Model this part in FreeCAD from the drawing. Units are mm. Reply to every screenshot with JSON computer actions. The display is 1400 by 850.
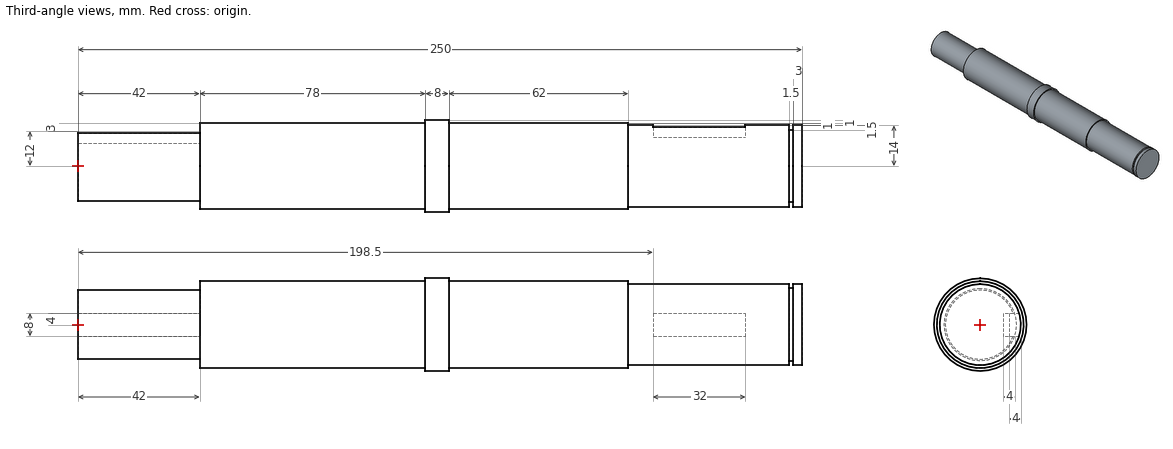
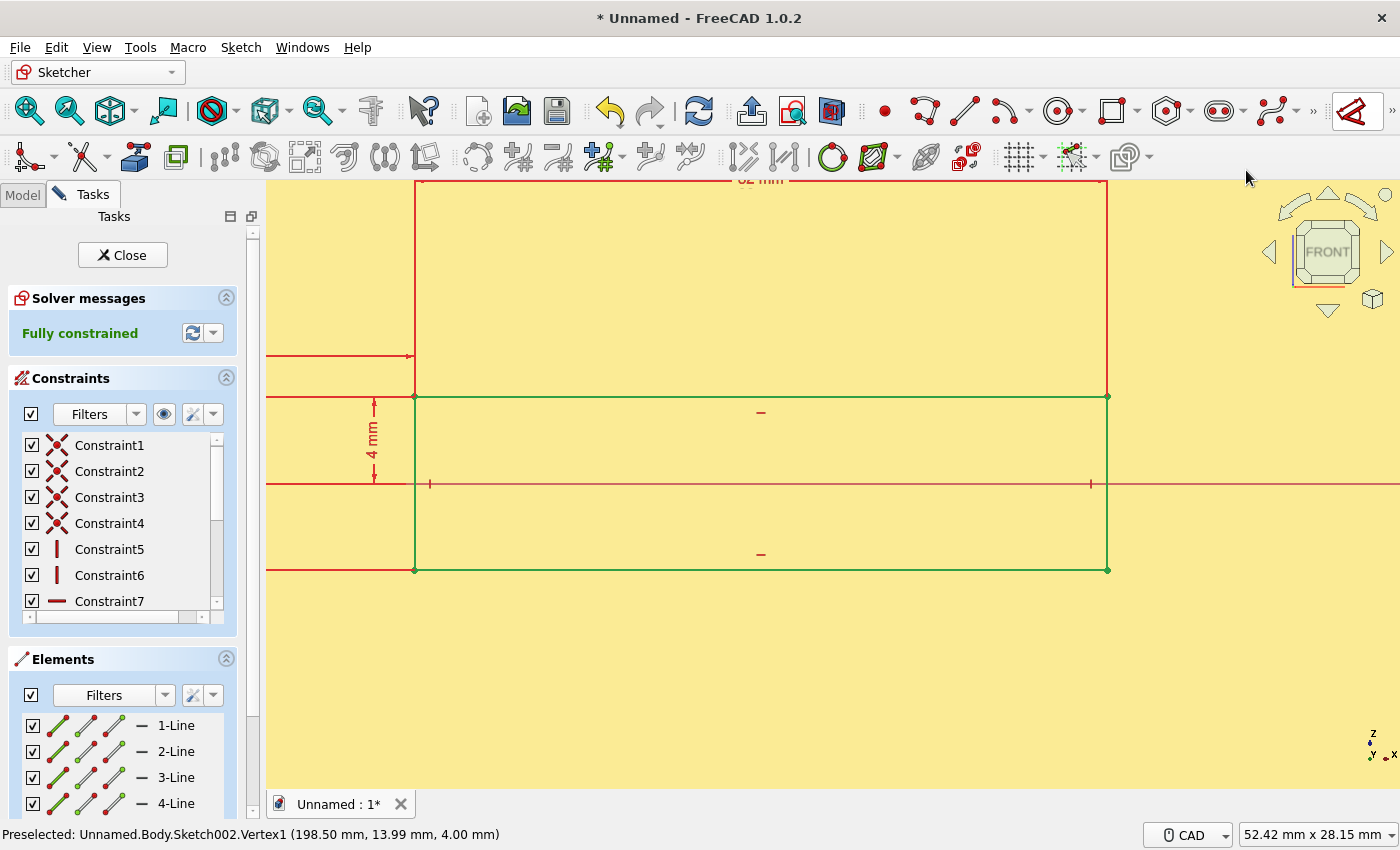
{"action": "left_click", "coordinate": [123, 255]}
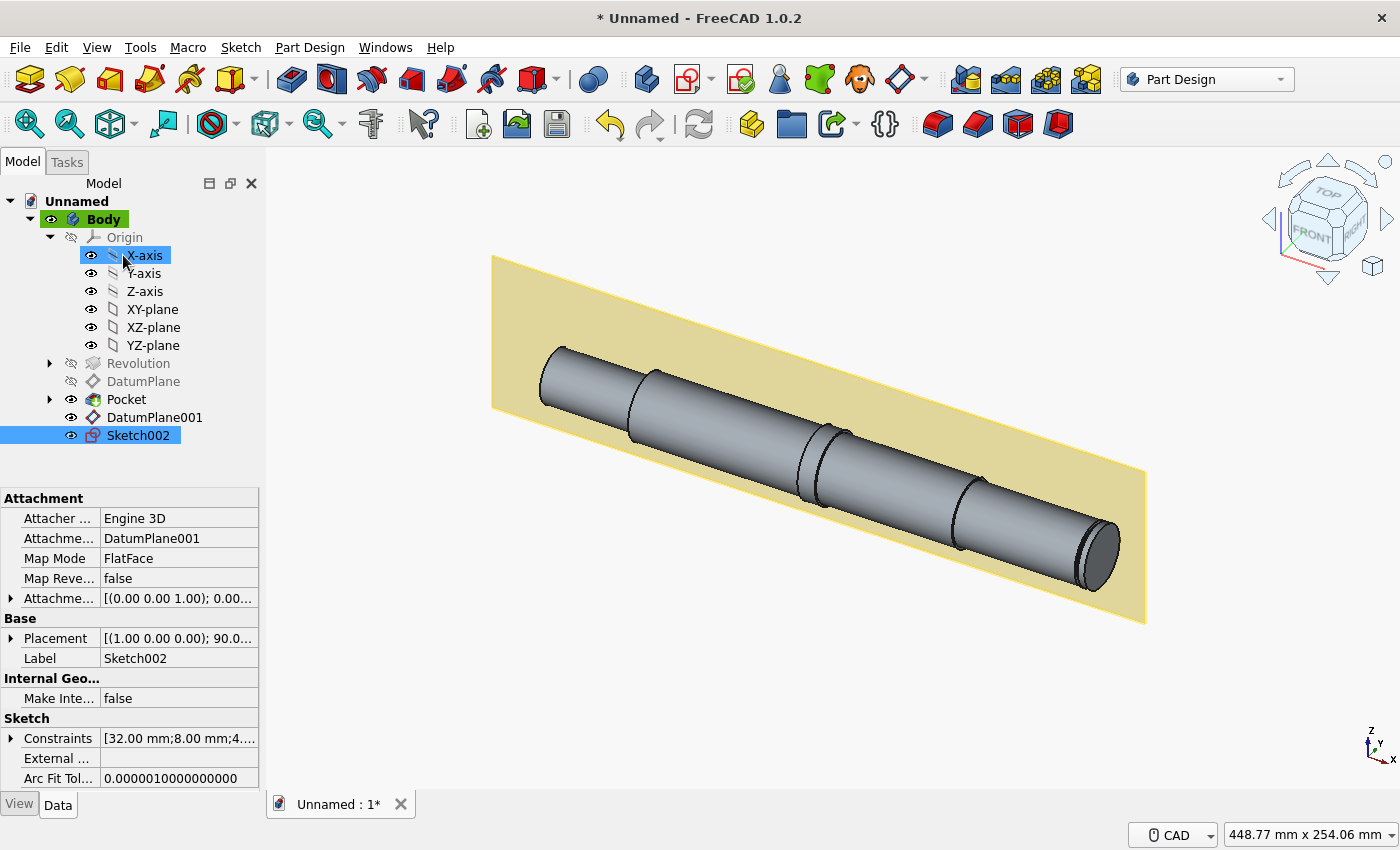
{"action": "left_click", "coordinate": [292, 80]}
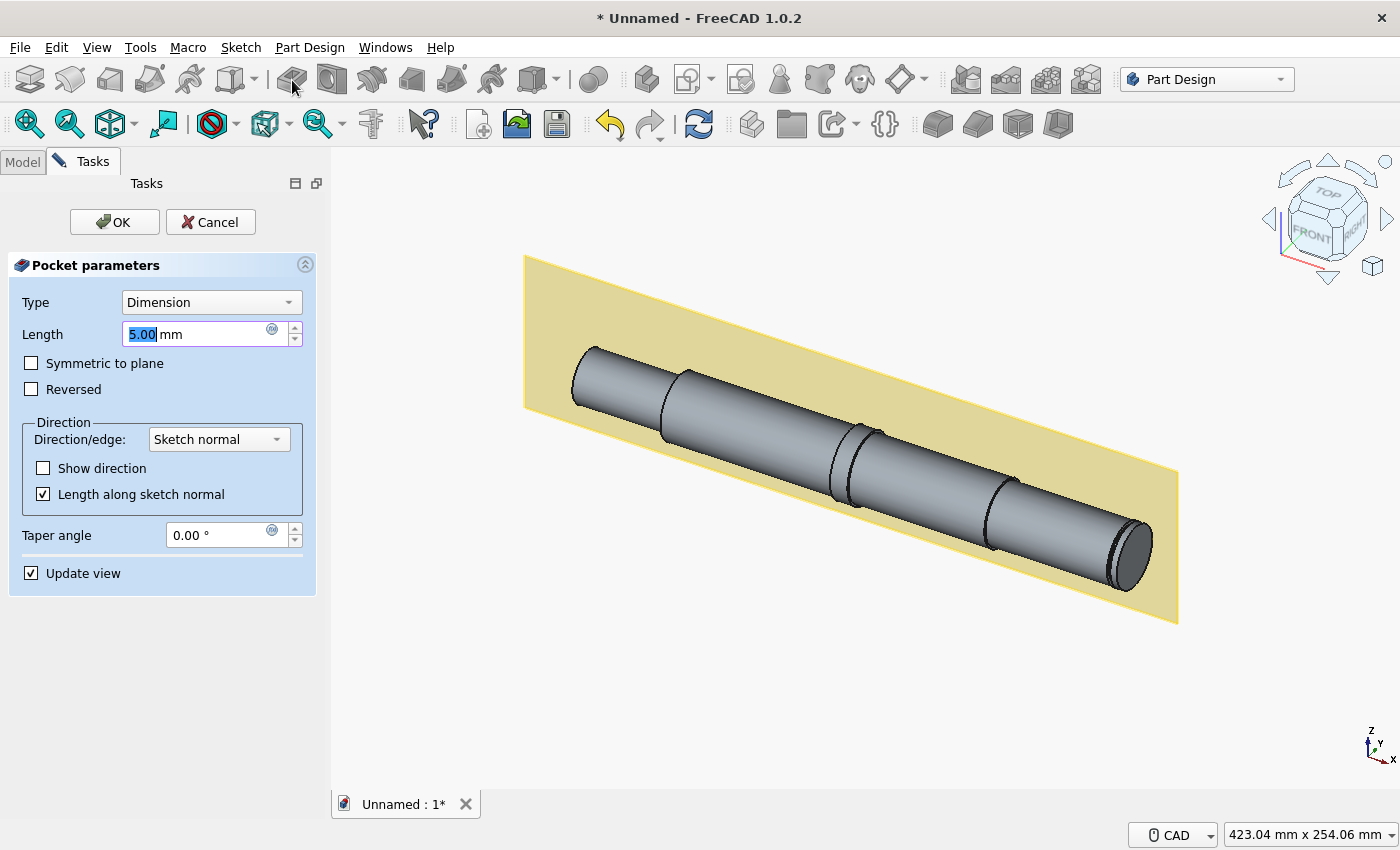
{"action": "type", "text": "4"}
{"action": "key", "text": "Tab"}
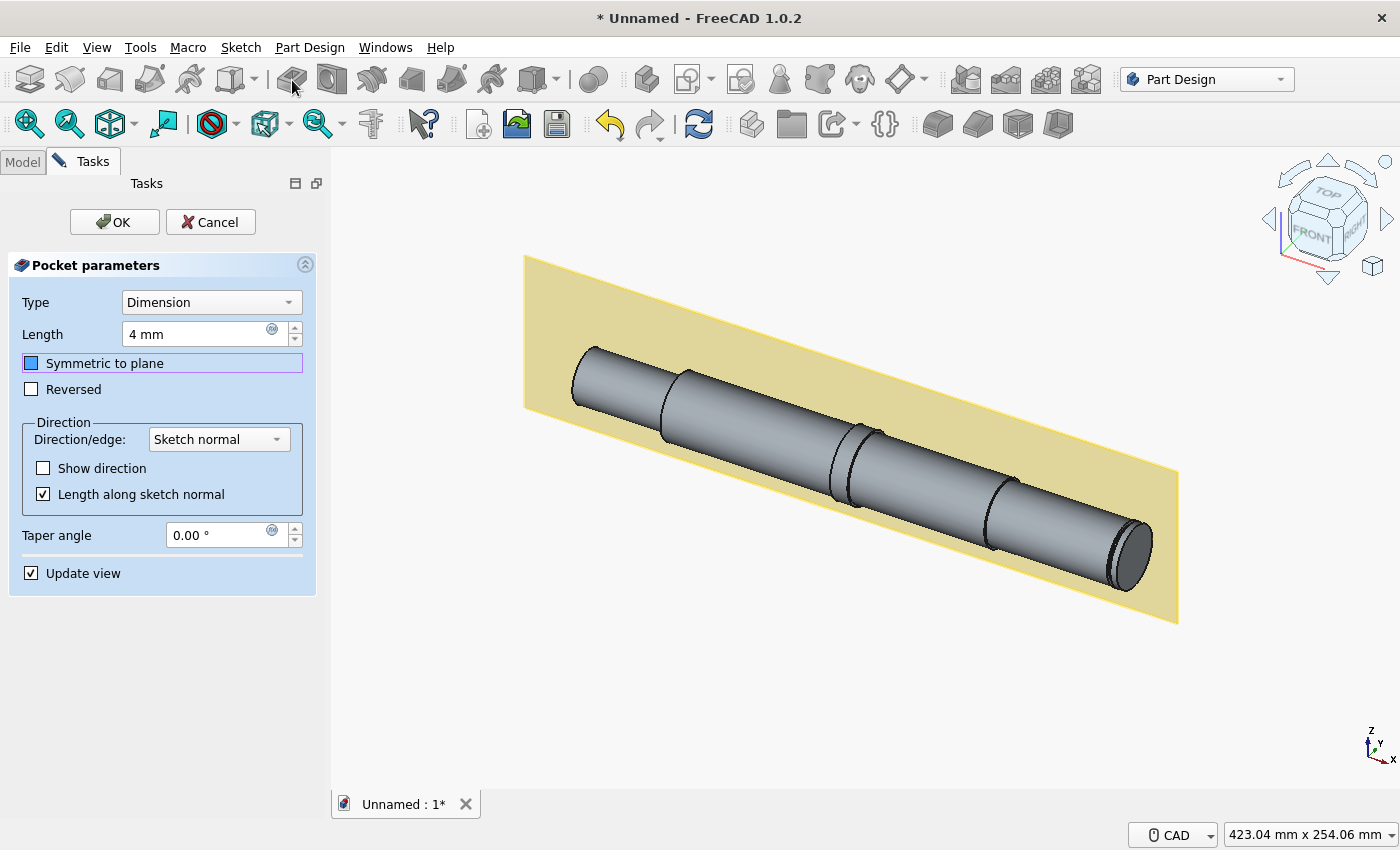
{"action": "left_click", "coordinate": [30, 389]}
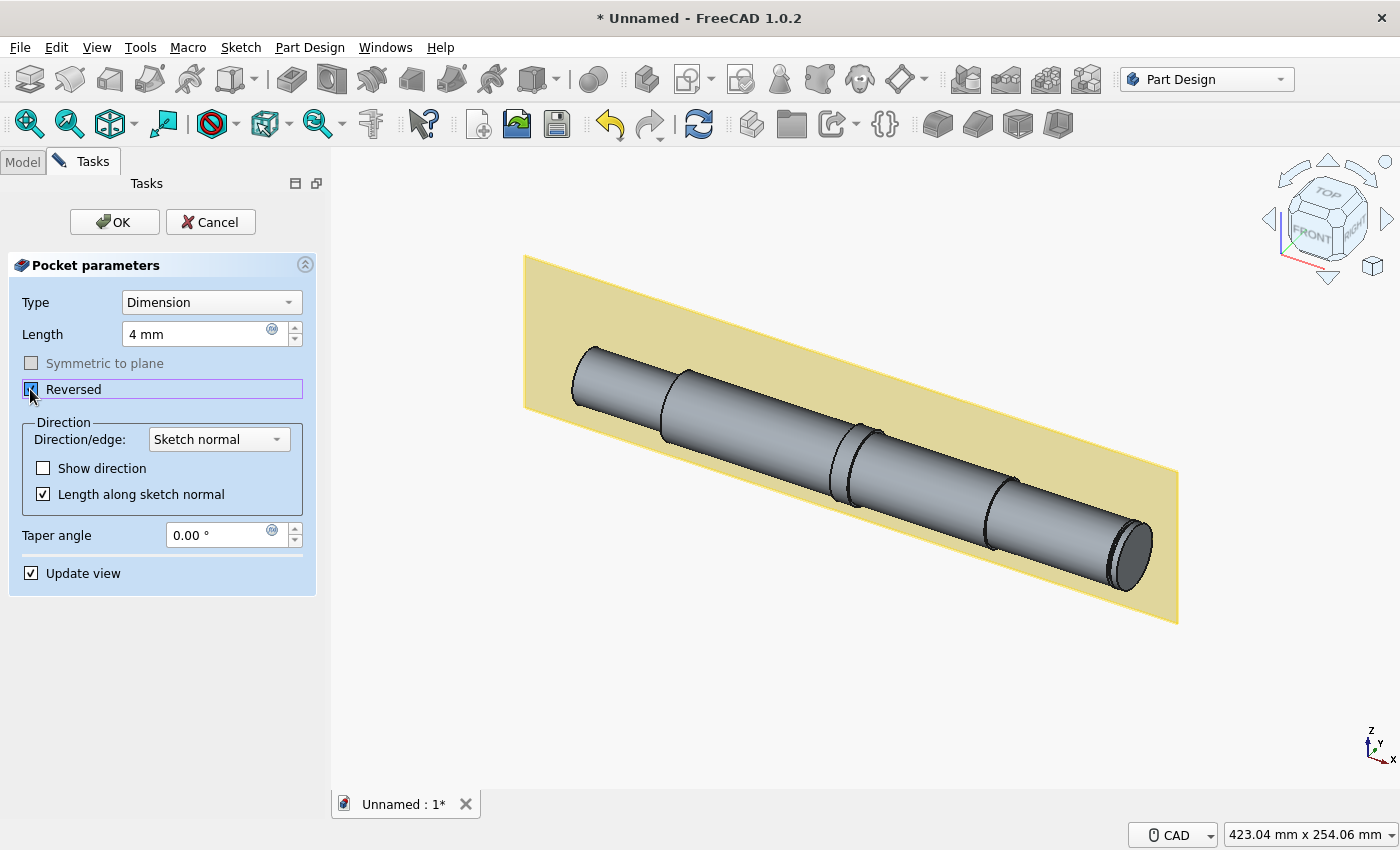
{"action": "left_click", "coordinate": [115, 222]}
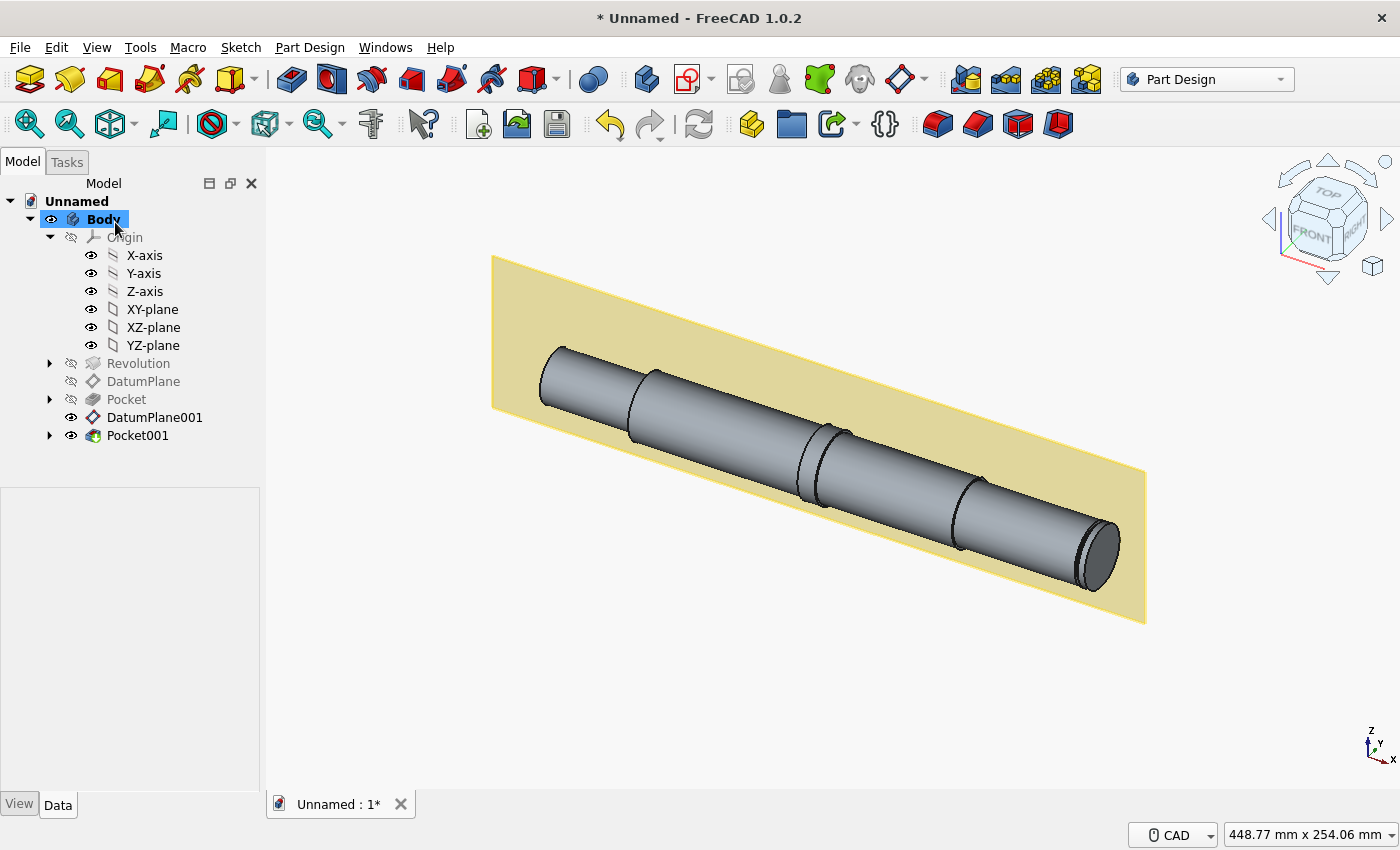
{"action": "left_click", "coordinate": [116, 417]}
{"action": "key", "text": "space"}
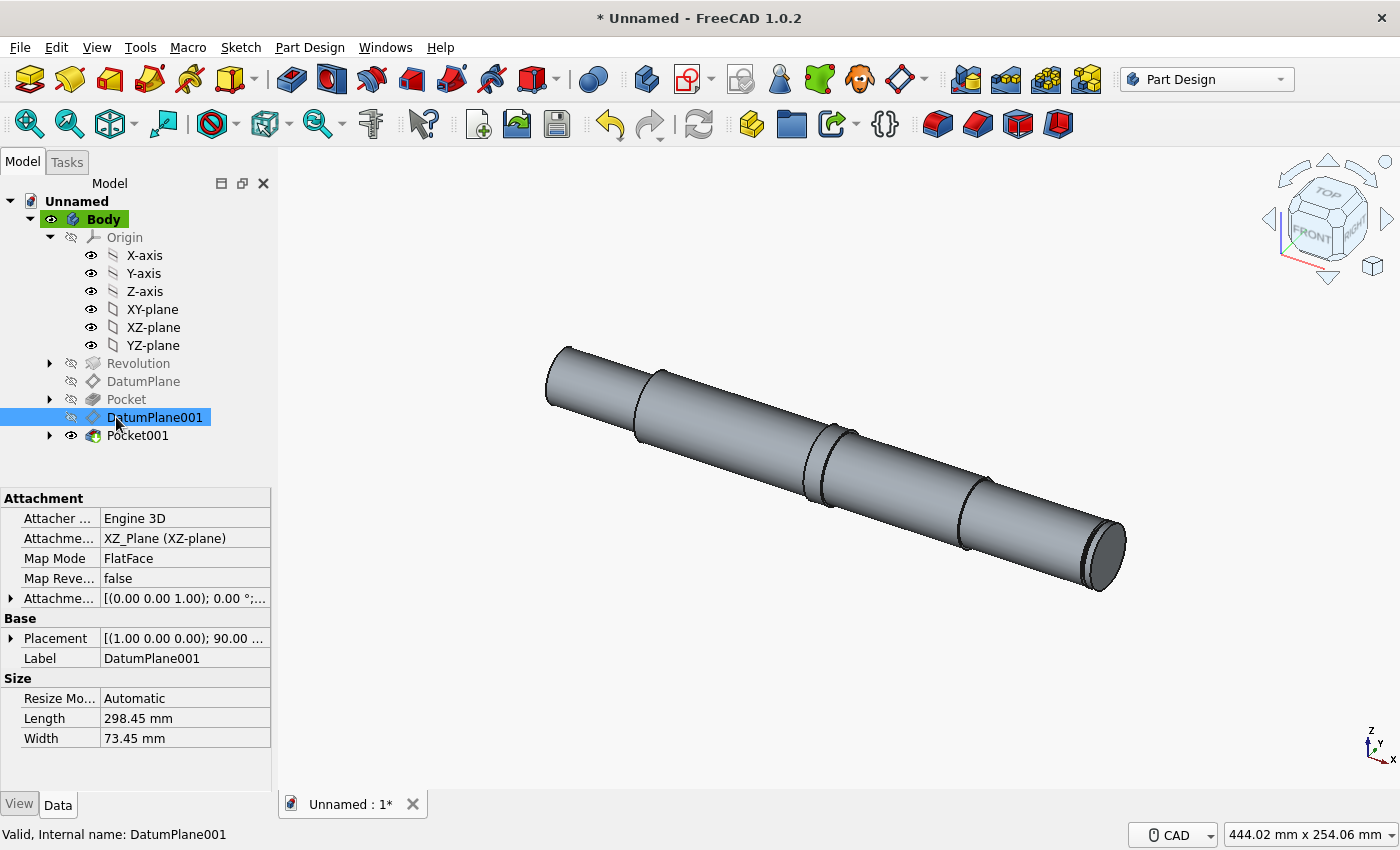
{"action": "key", "text": "0"}